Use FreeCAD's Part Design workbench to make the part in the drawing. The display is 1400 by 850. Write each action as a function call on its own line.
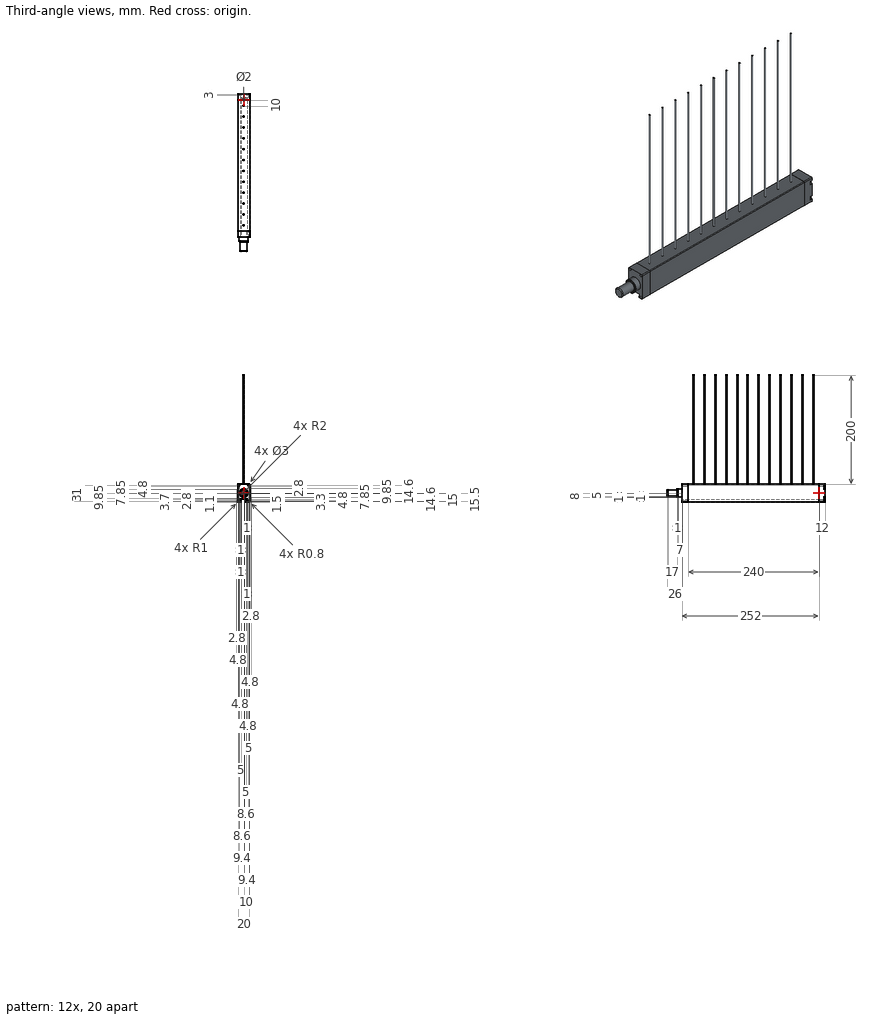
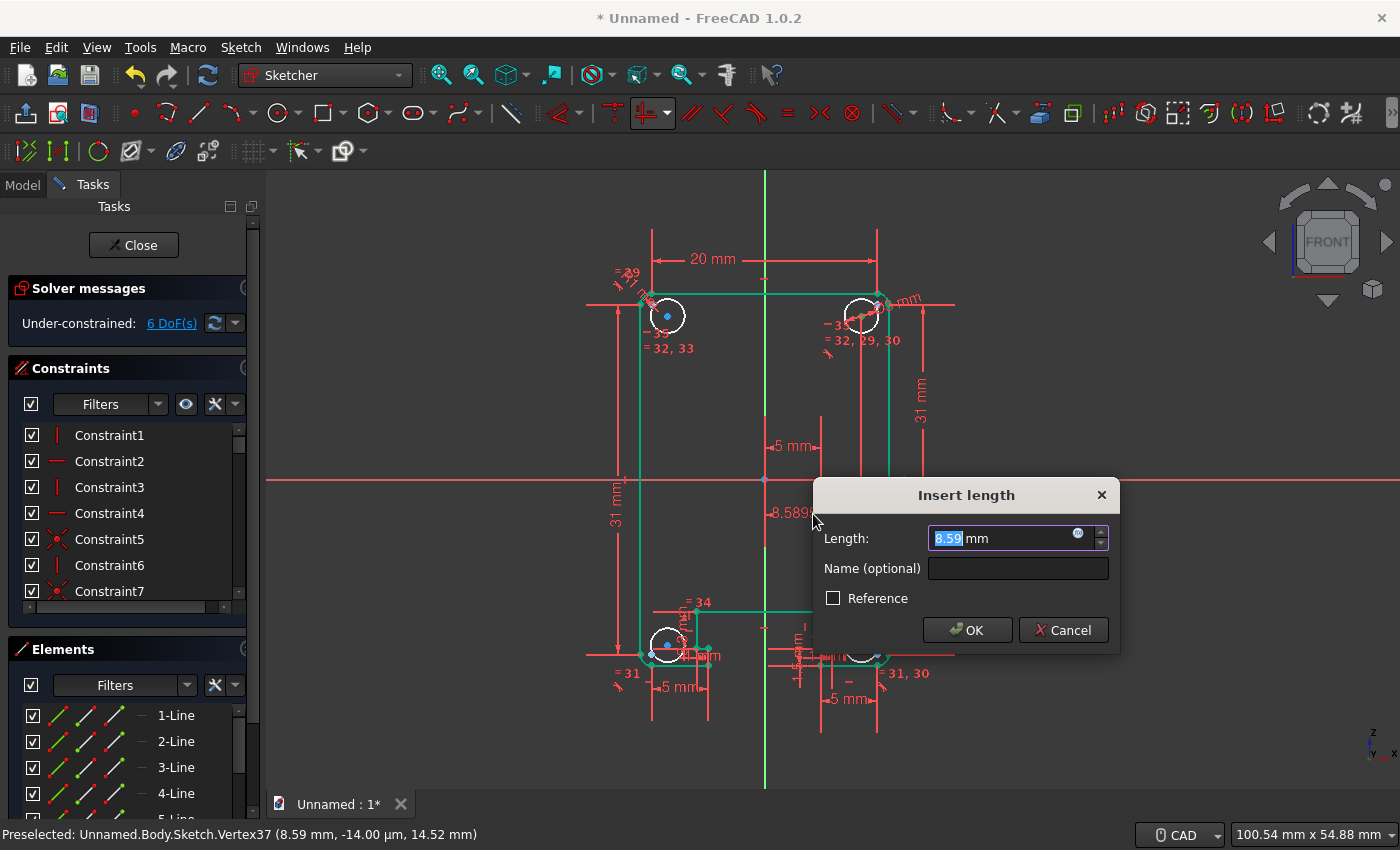
text(8.6)
key(Return)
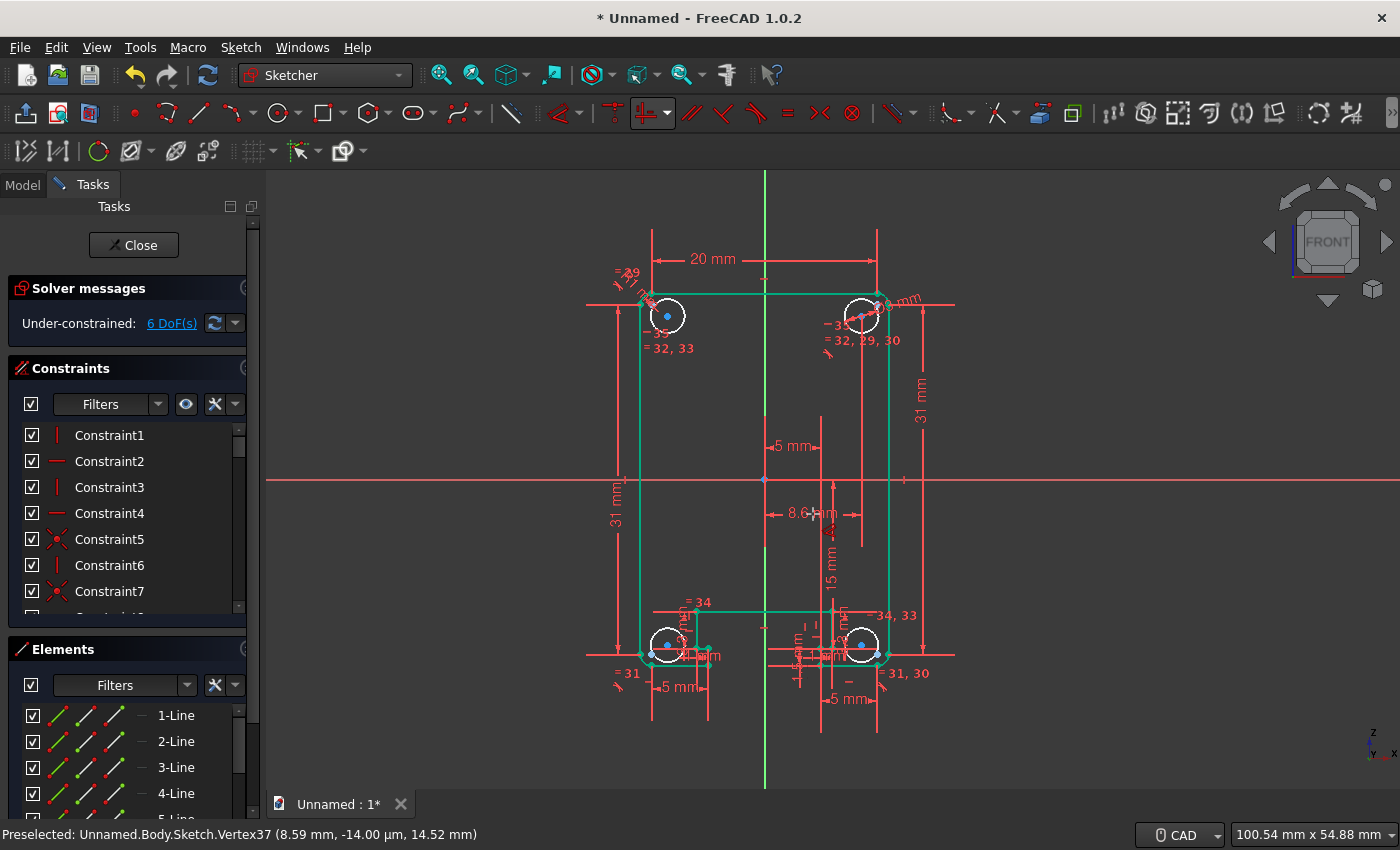
click(668, 316)
click(716, 514)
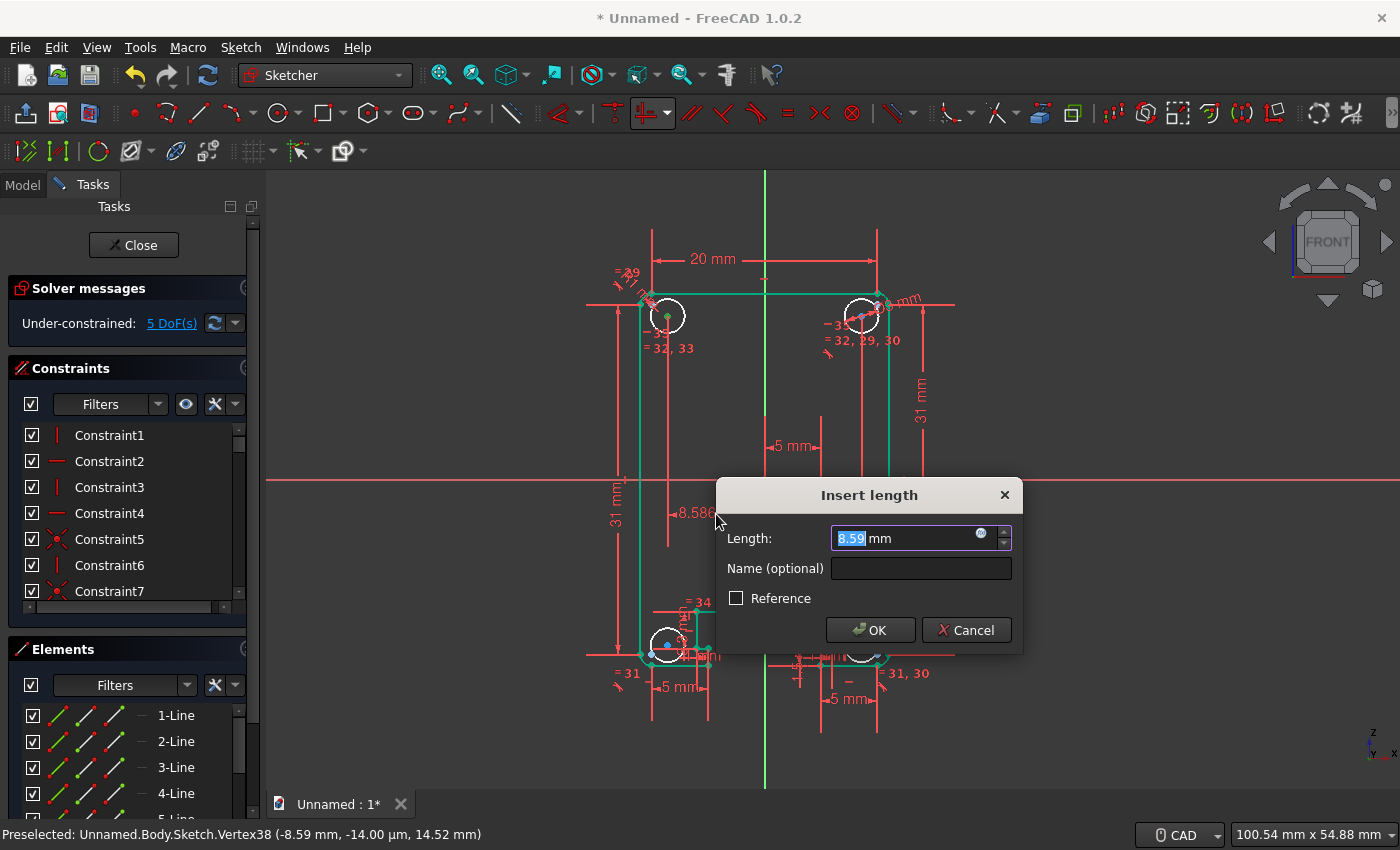
text(8.6)
key(Return)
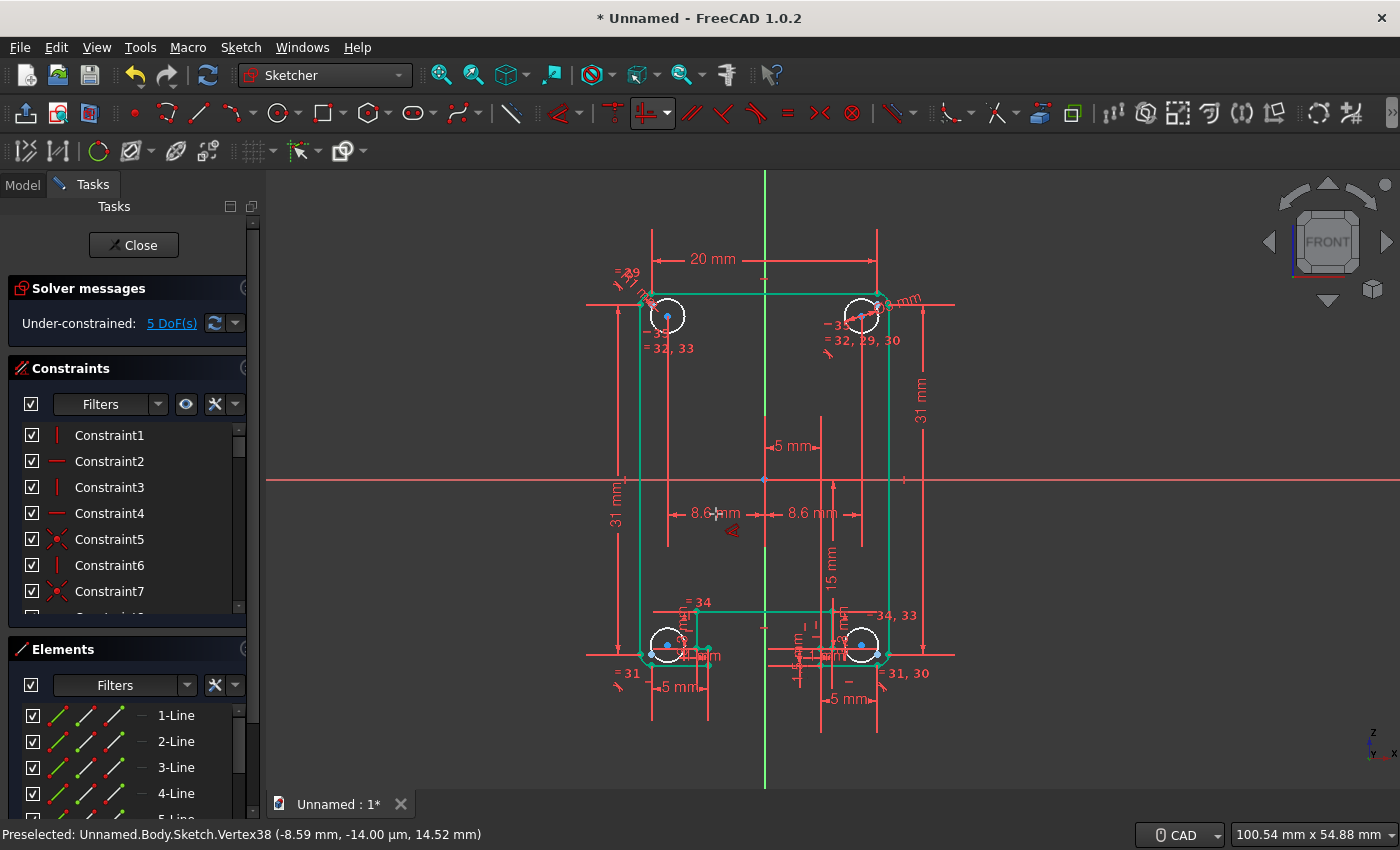
click(861, 645)
click(813, 679)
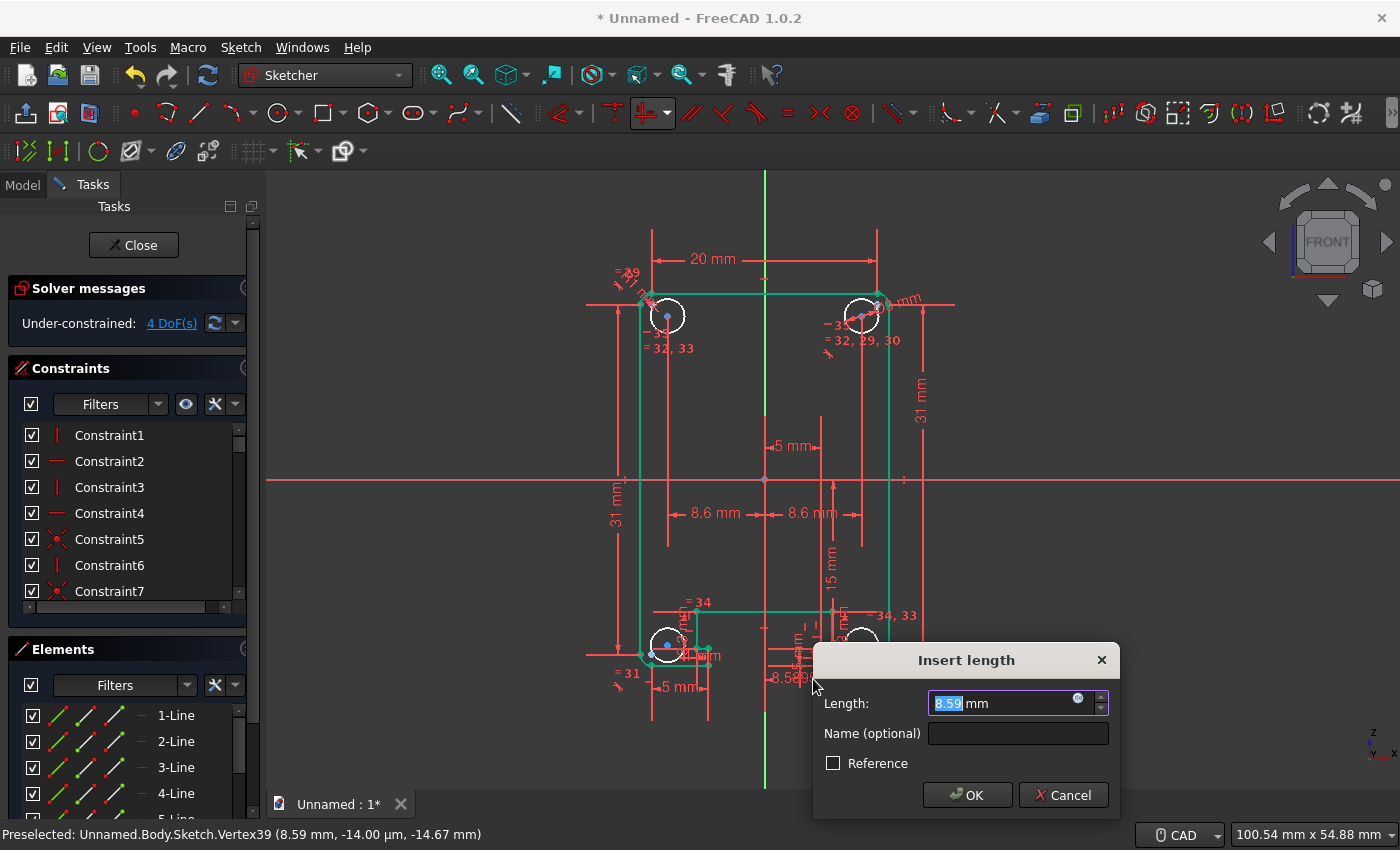
text(8.6)
key(Return)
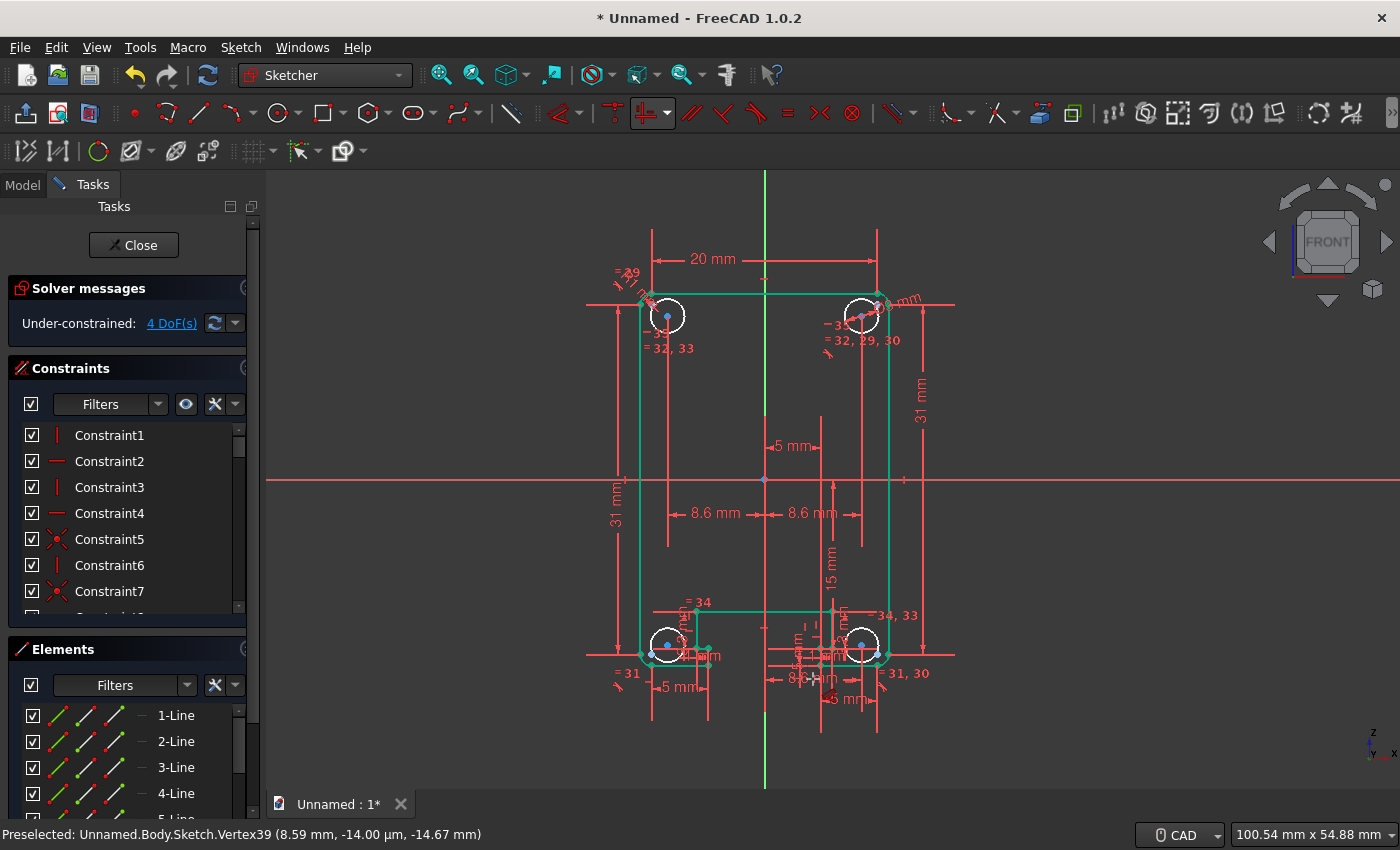
click(668, 645)
click(716, 446)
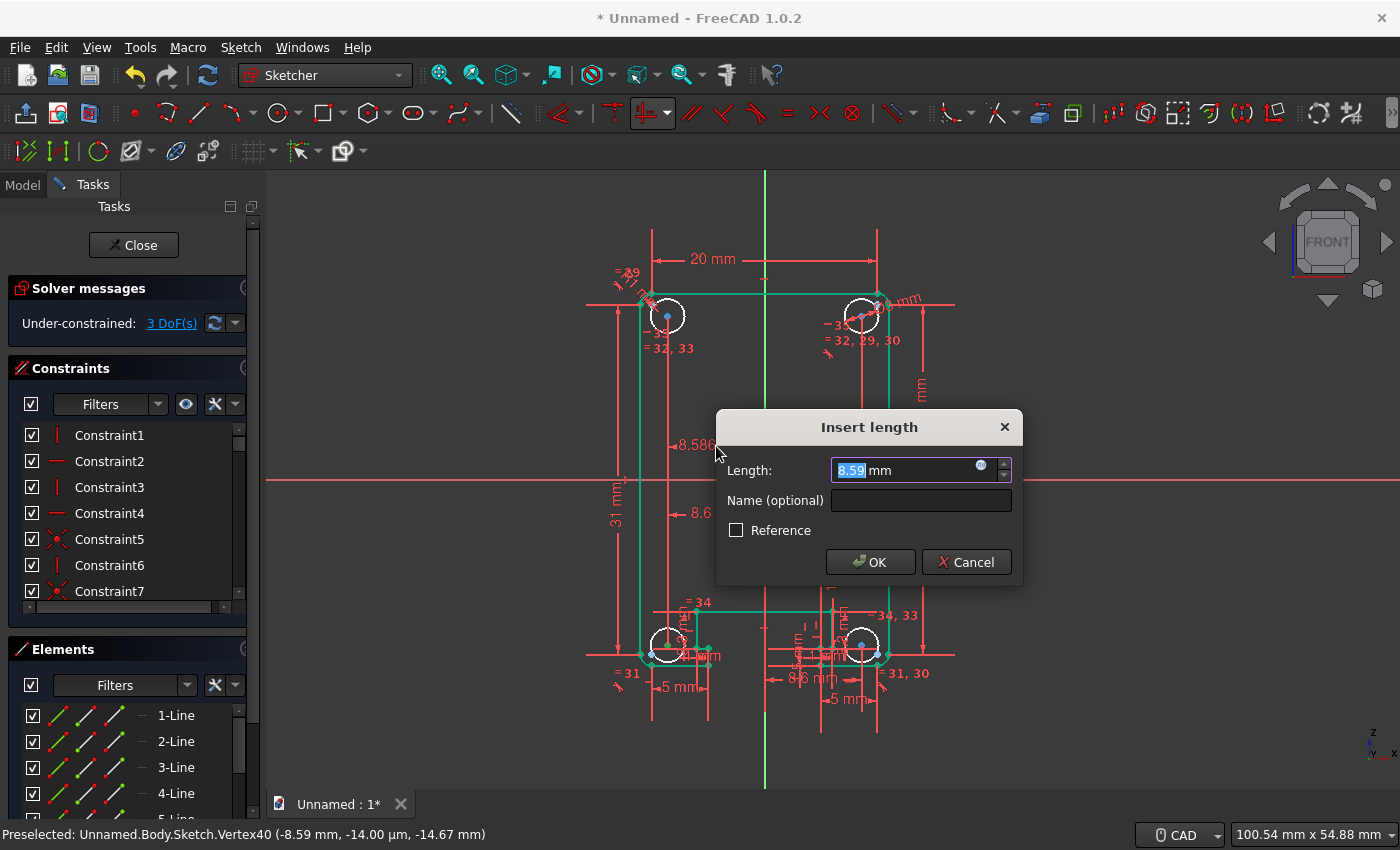
text(8.6)
key(Return)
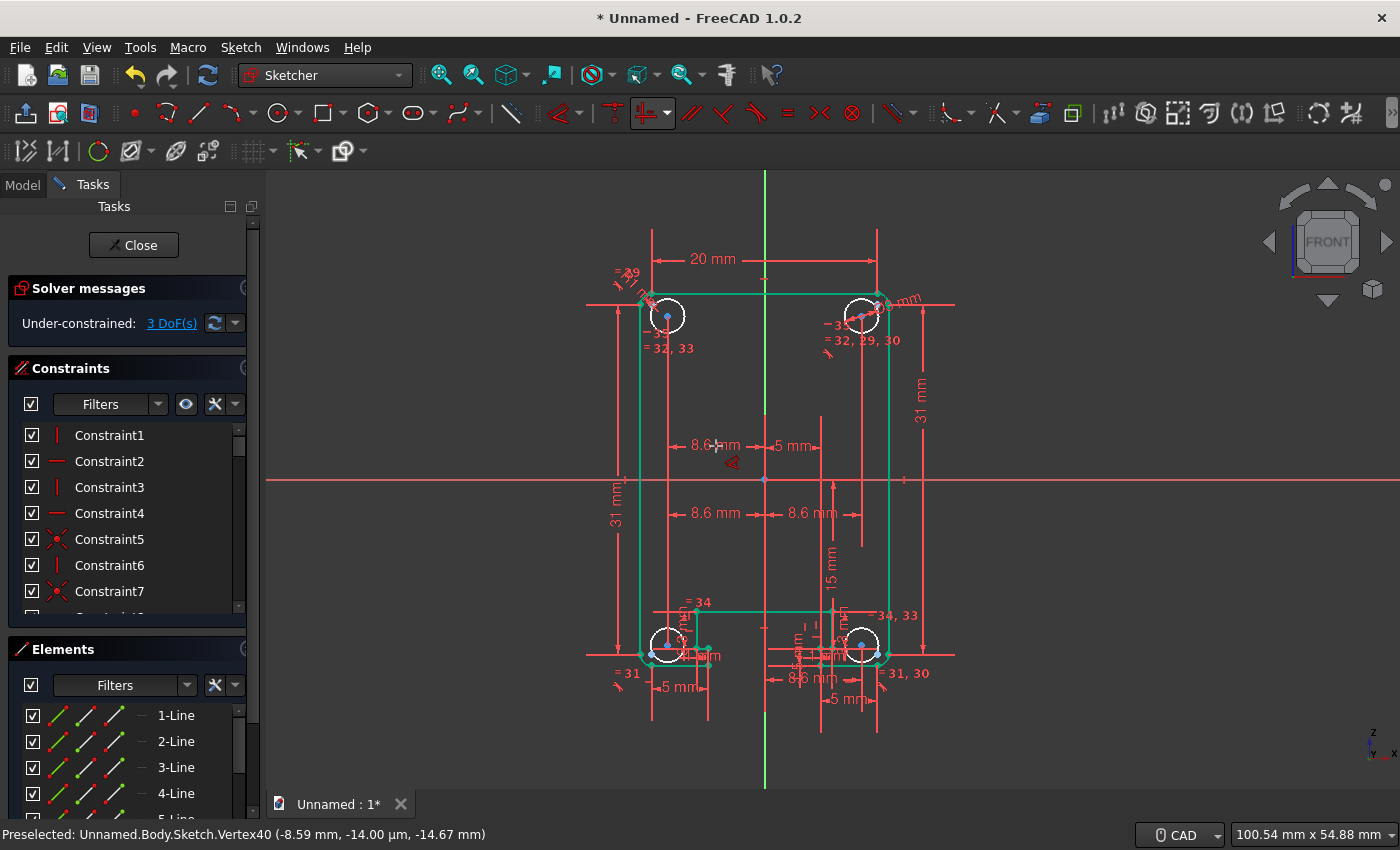
click(862, 316)
click(731, 398)